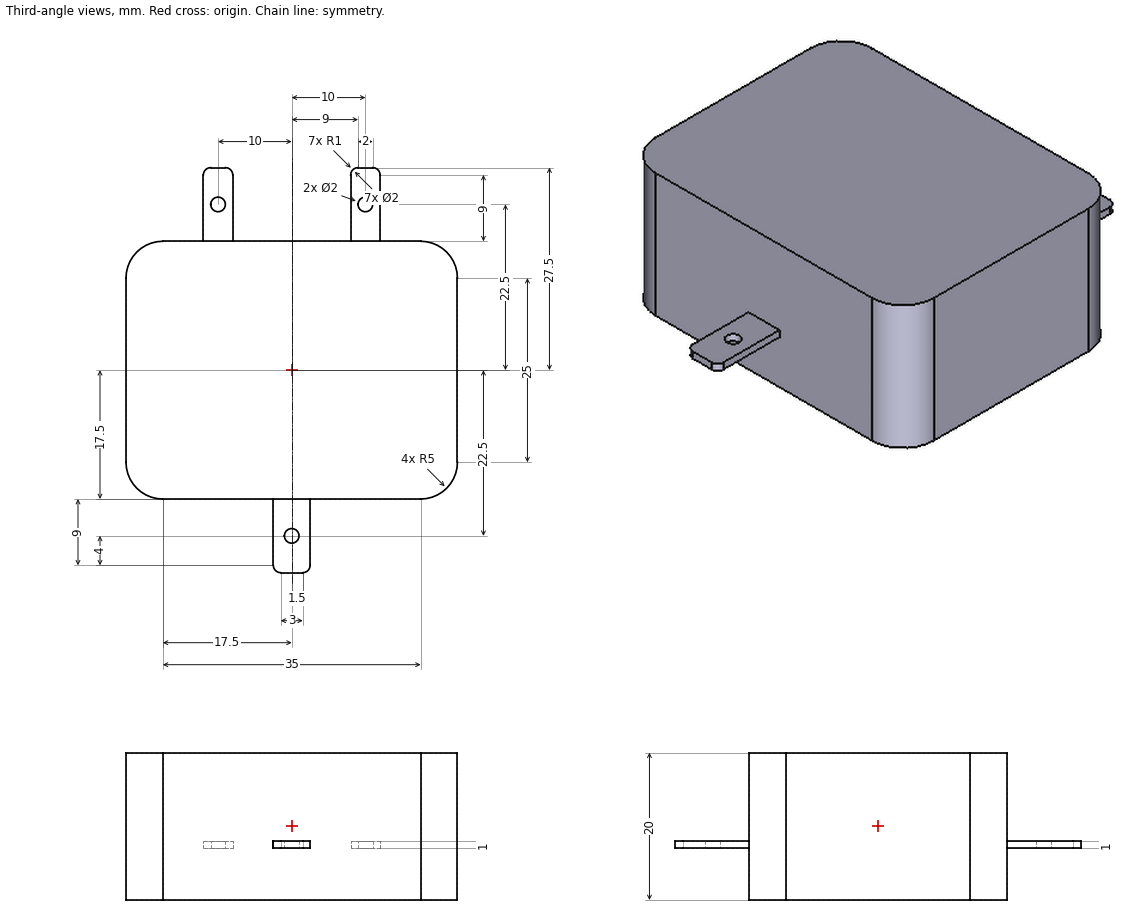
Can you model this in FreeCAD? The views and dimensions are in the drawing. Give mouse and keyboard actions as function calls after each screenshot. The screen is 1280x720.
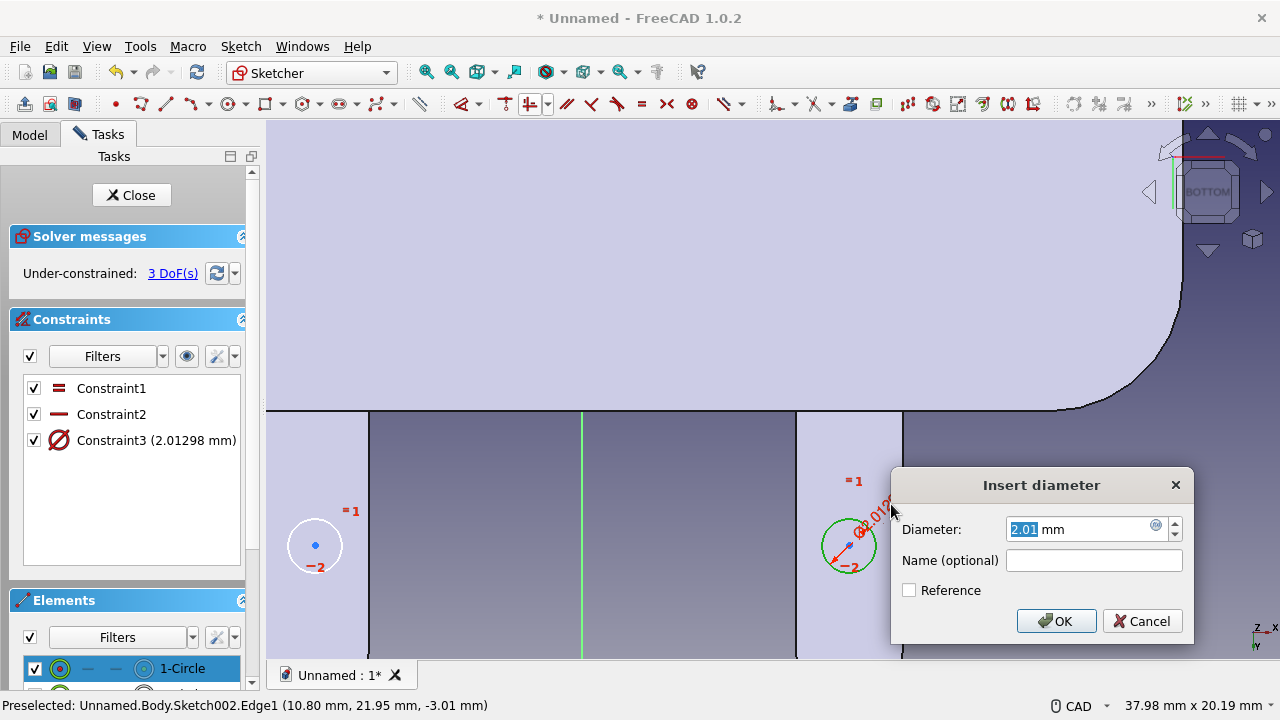
text(2)
key(Return)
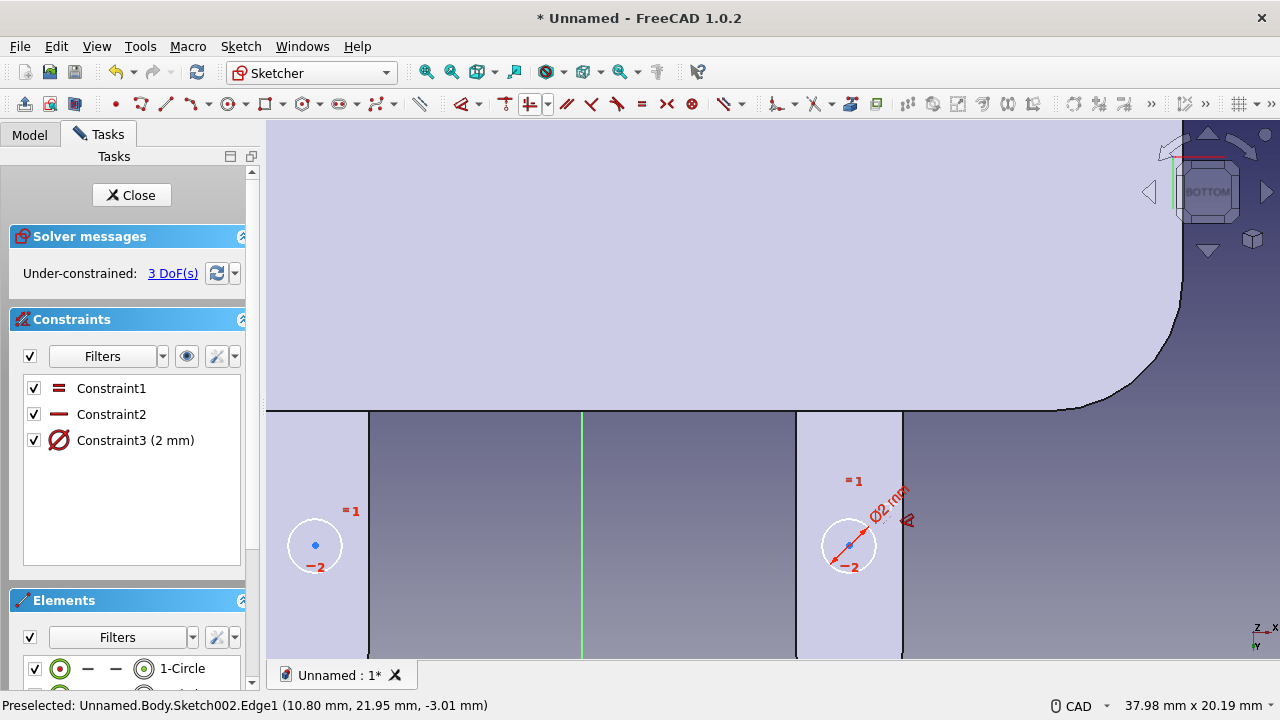
click(849, 546)
click(716, 580)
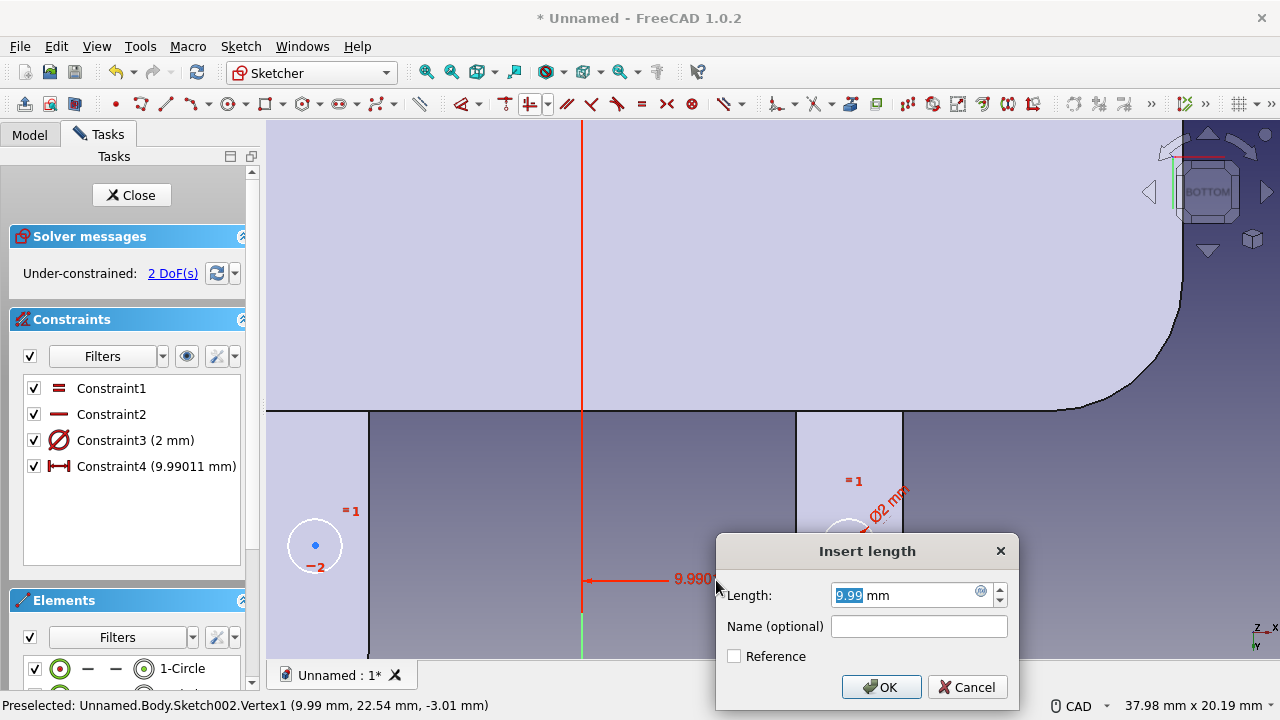
text(10)
key(Return)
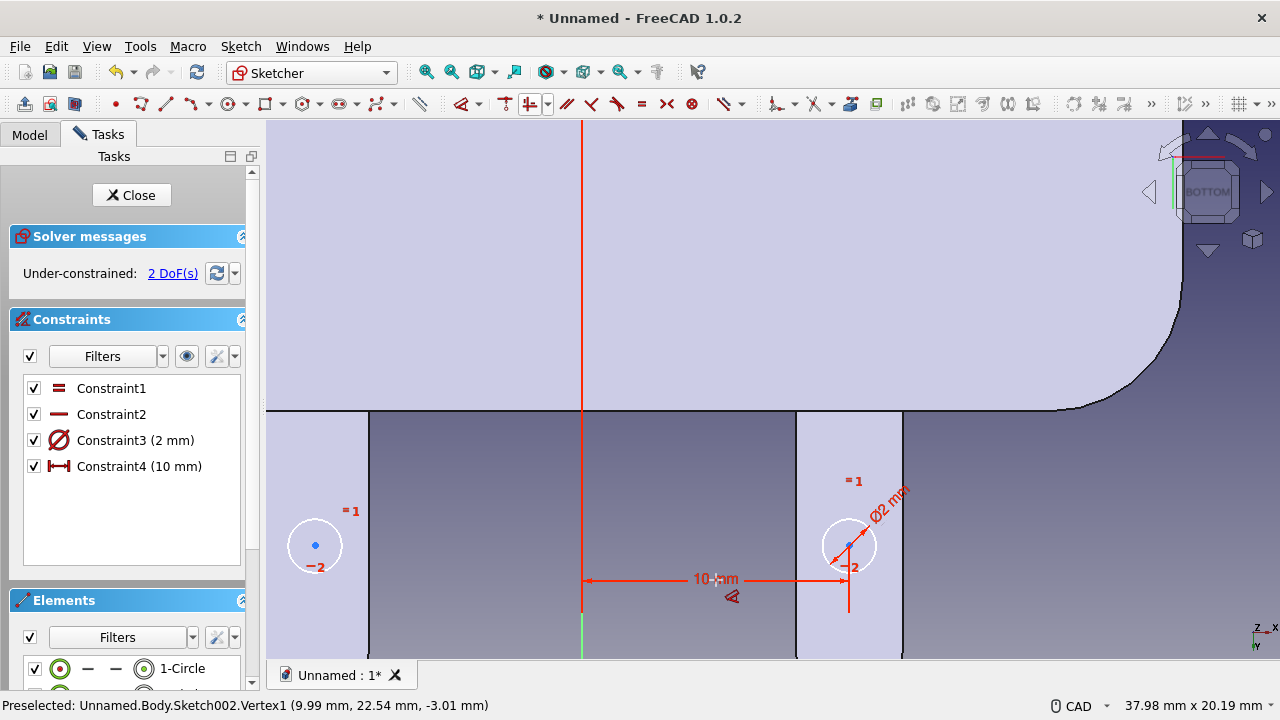
click(315, 546)
click(449, 580)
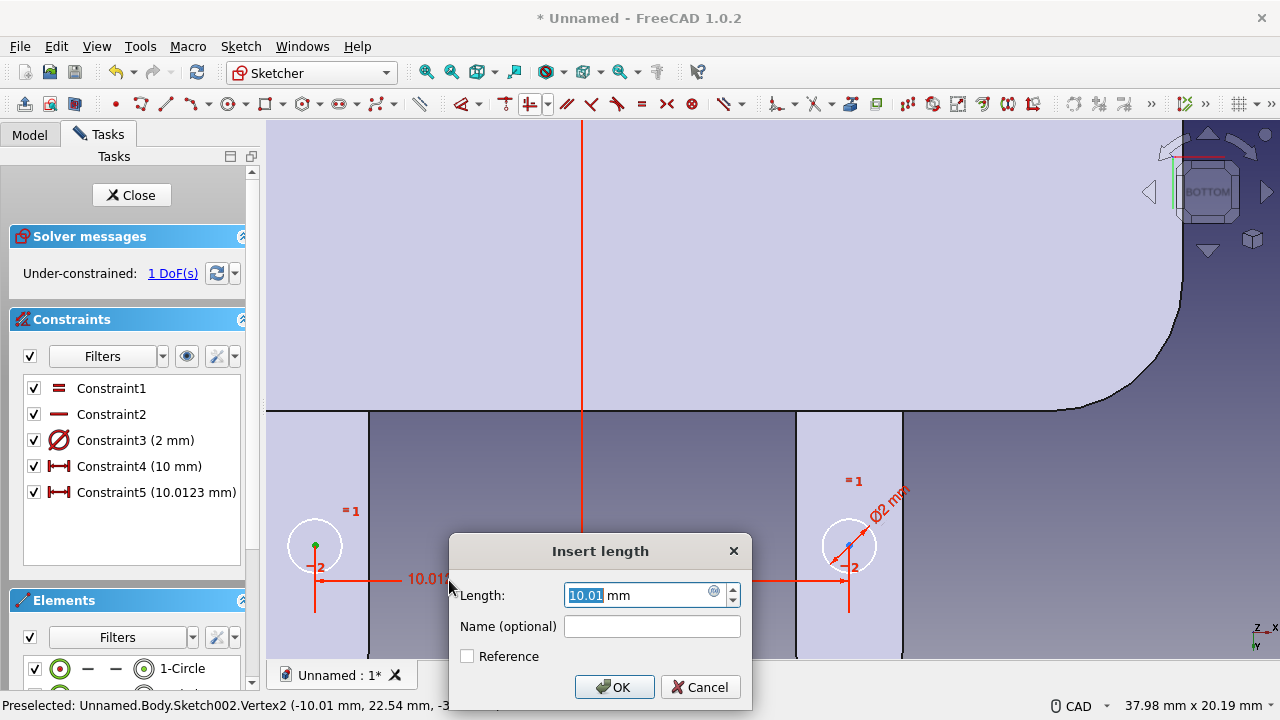
text(10)
key(Return)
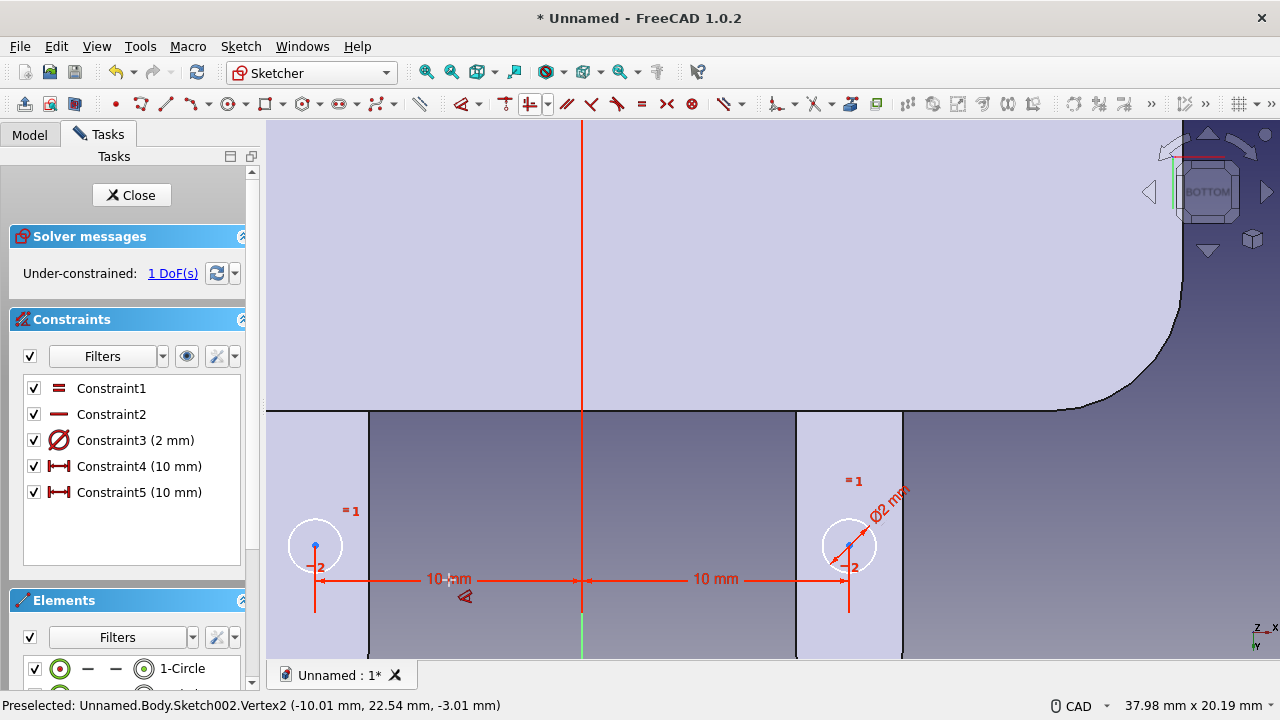
click(849, 546)
click(883, 347)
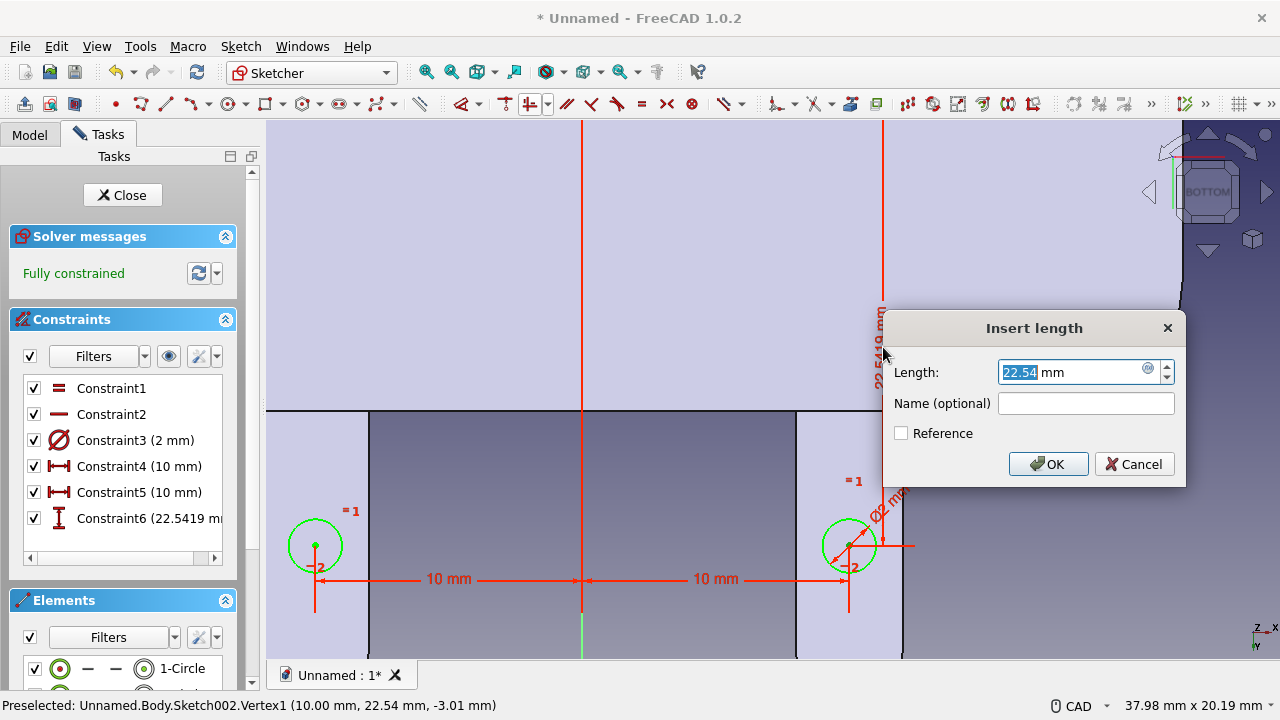
text(22.5)
key(Return)
key(Escape)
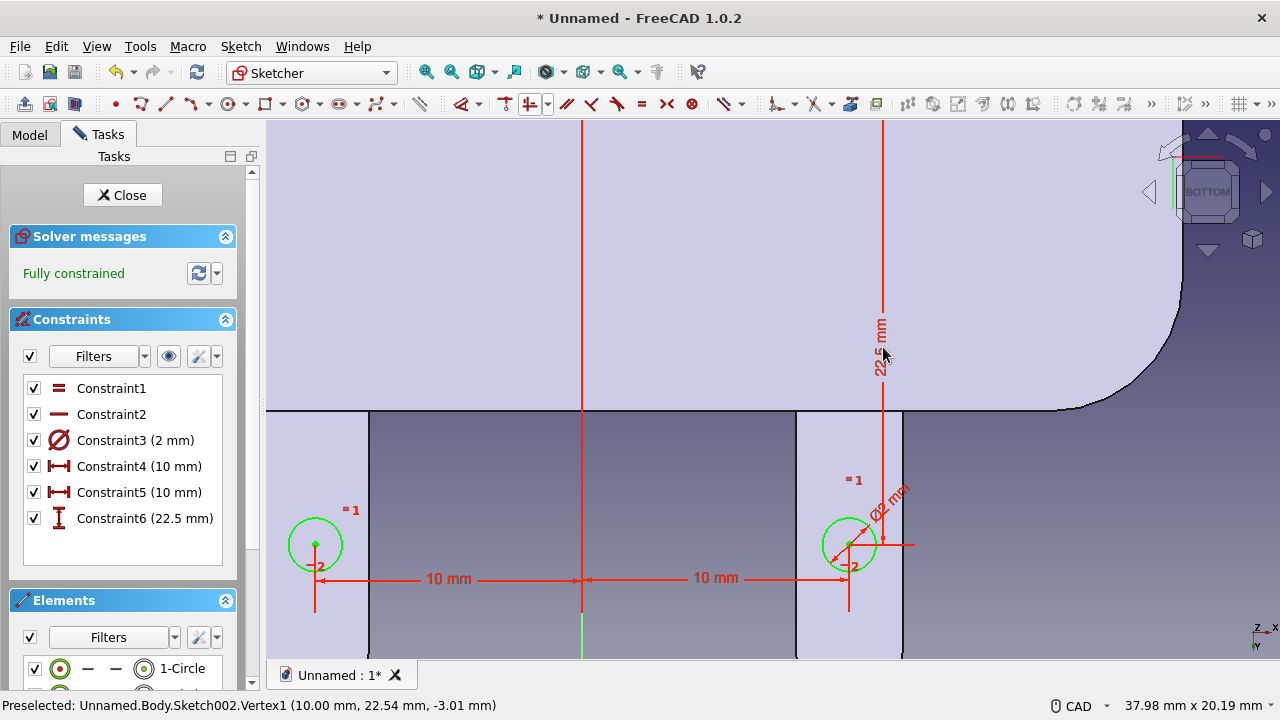
click(123, 195)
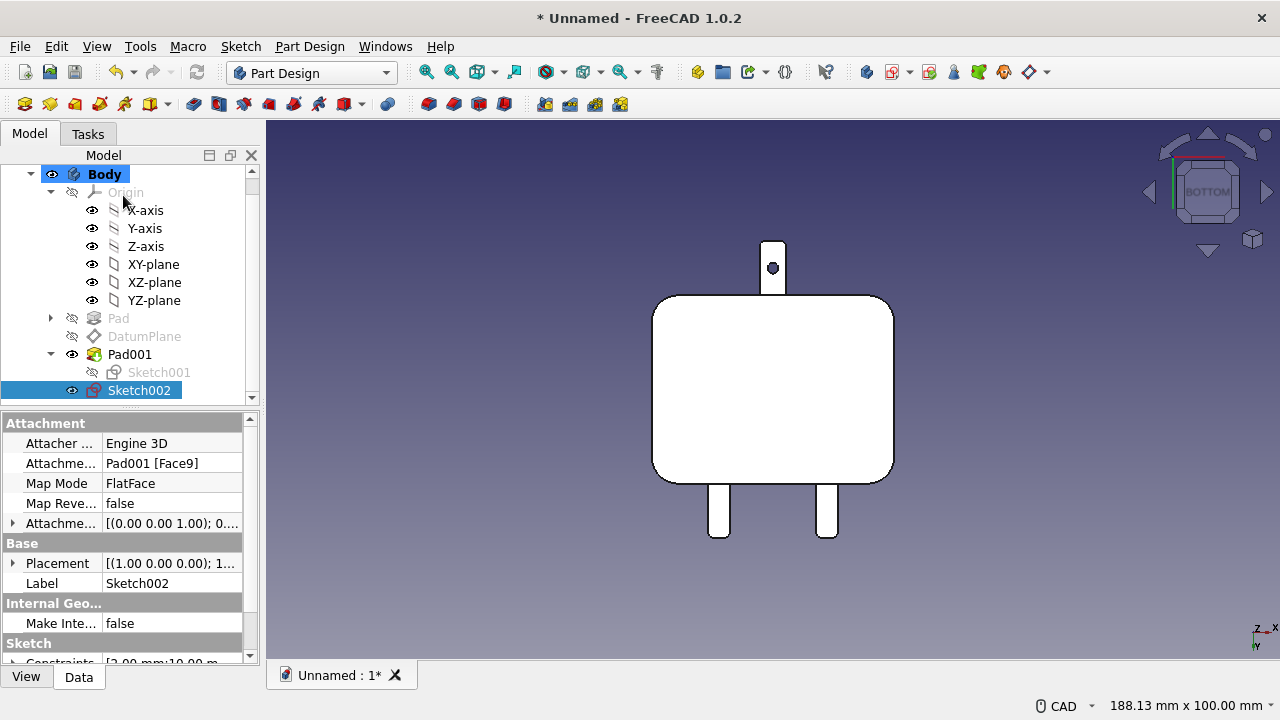
click(194, 104)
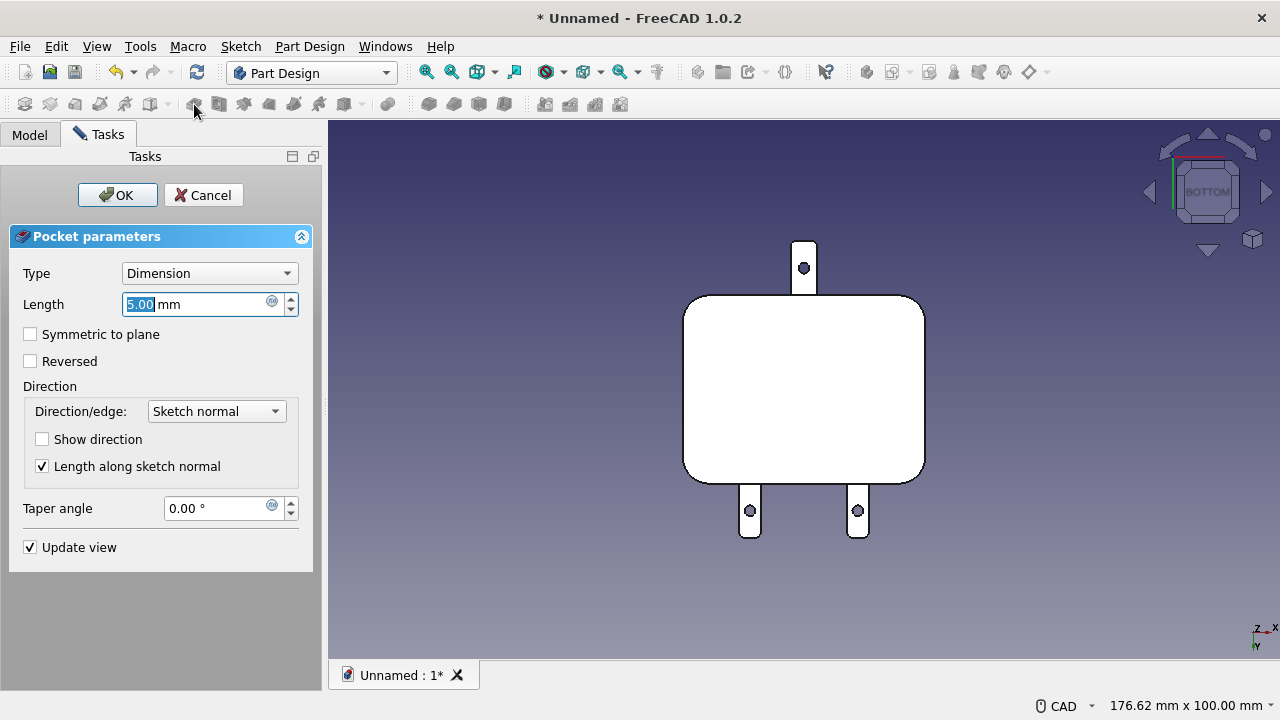
text(1)
key(Tab)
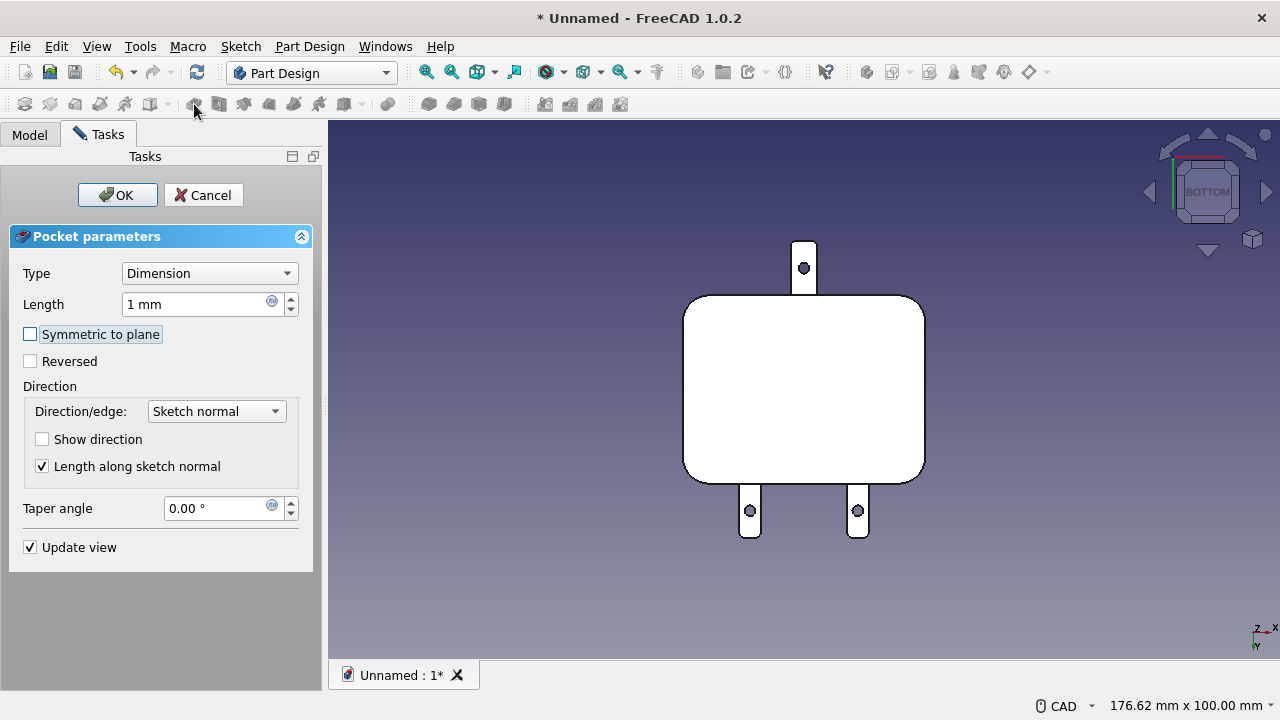
click(118, 195)